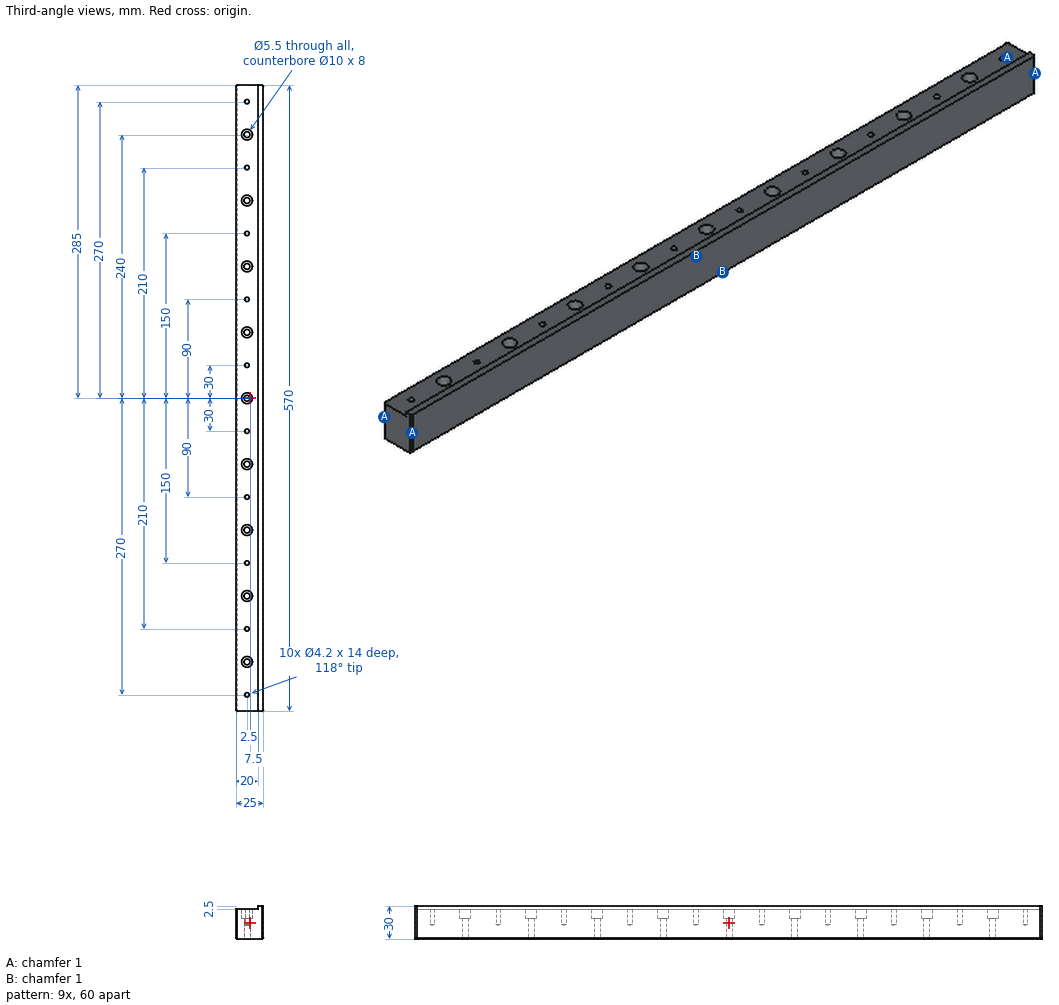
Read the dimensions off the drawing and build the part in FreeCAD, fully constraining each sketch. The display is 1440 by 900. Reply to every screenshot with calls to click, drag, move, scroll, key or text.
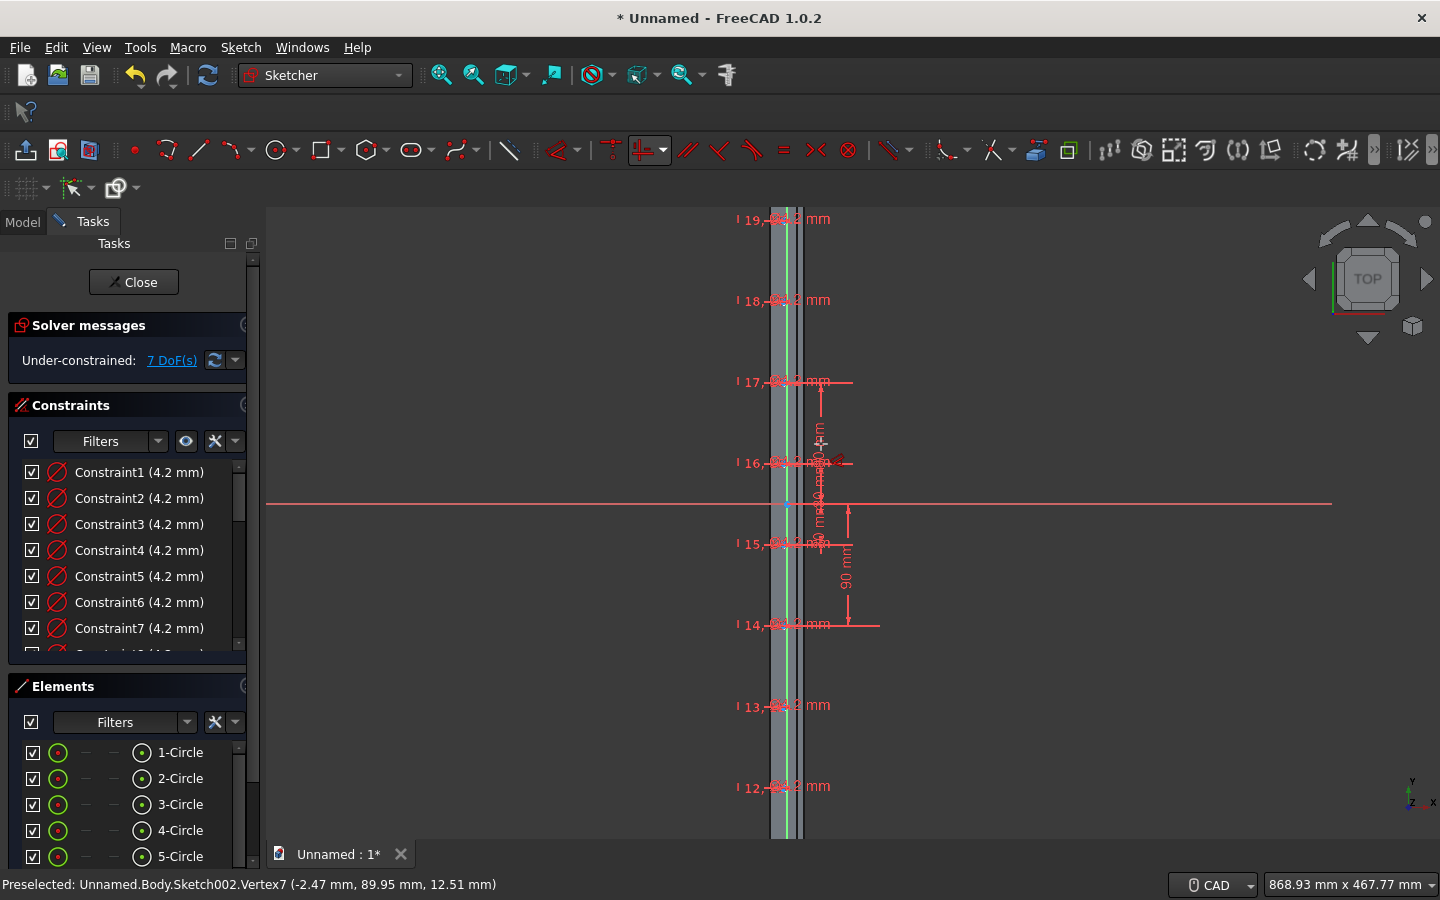
scroll(785, 546, down, 3)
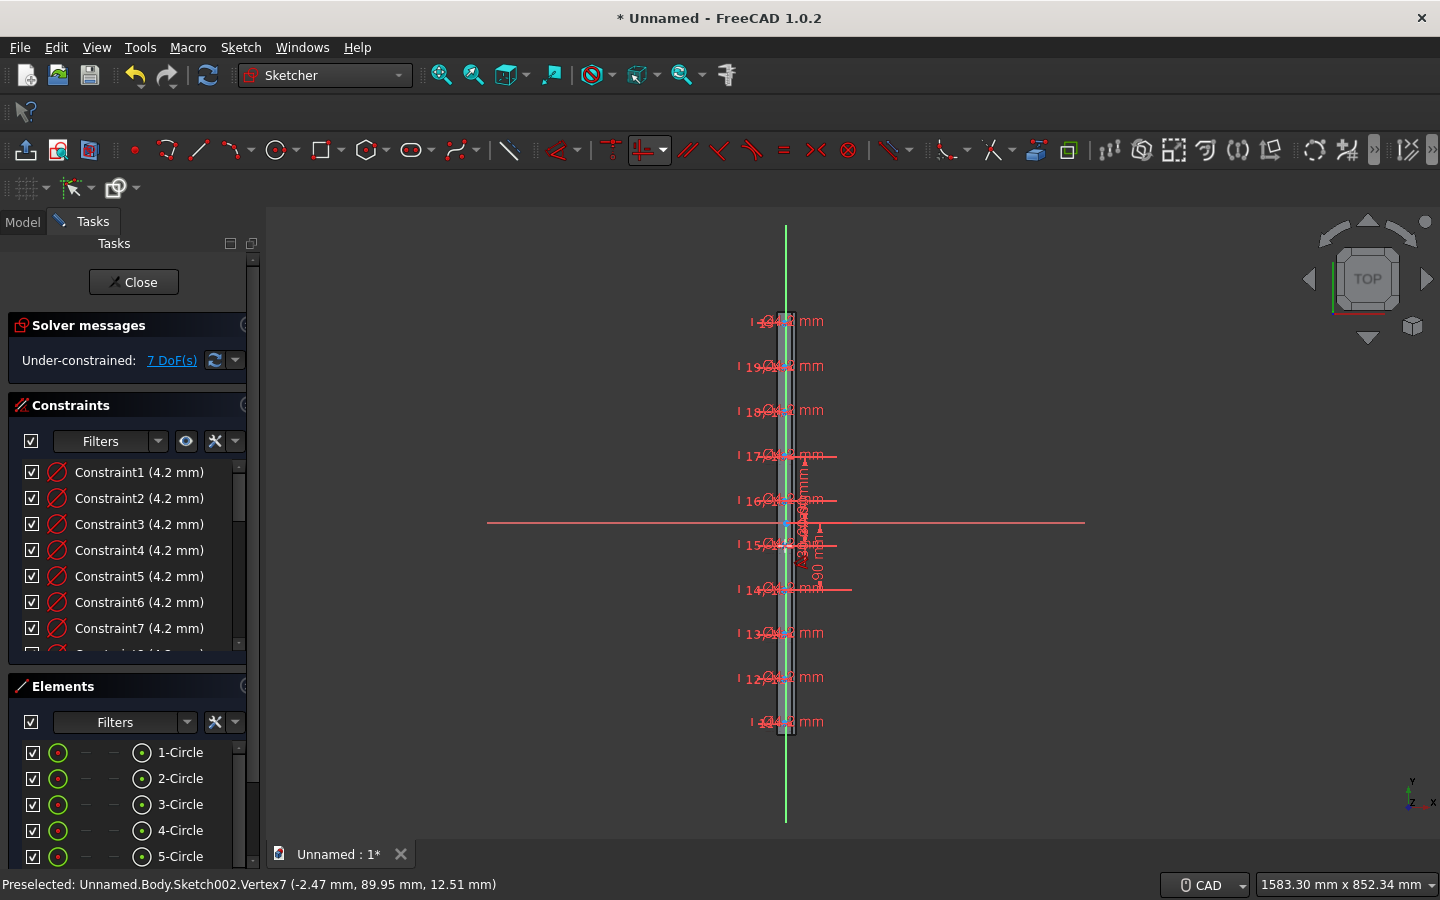
scroll(785, 724, up, 16)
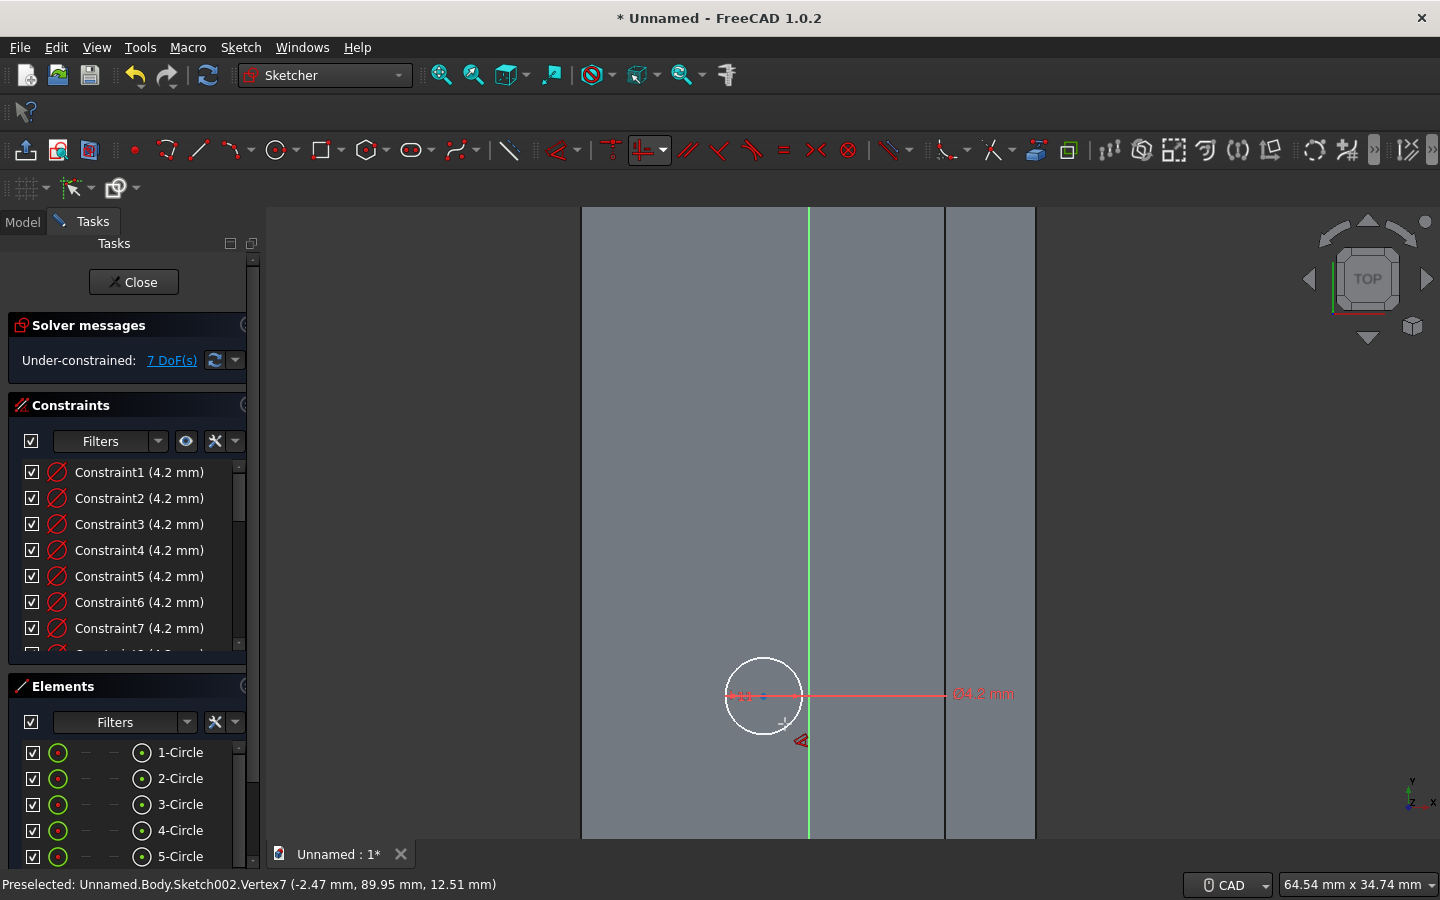
click(764, 696)
click(786, 754)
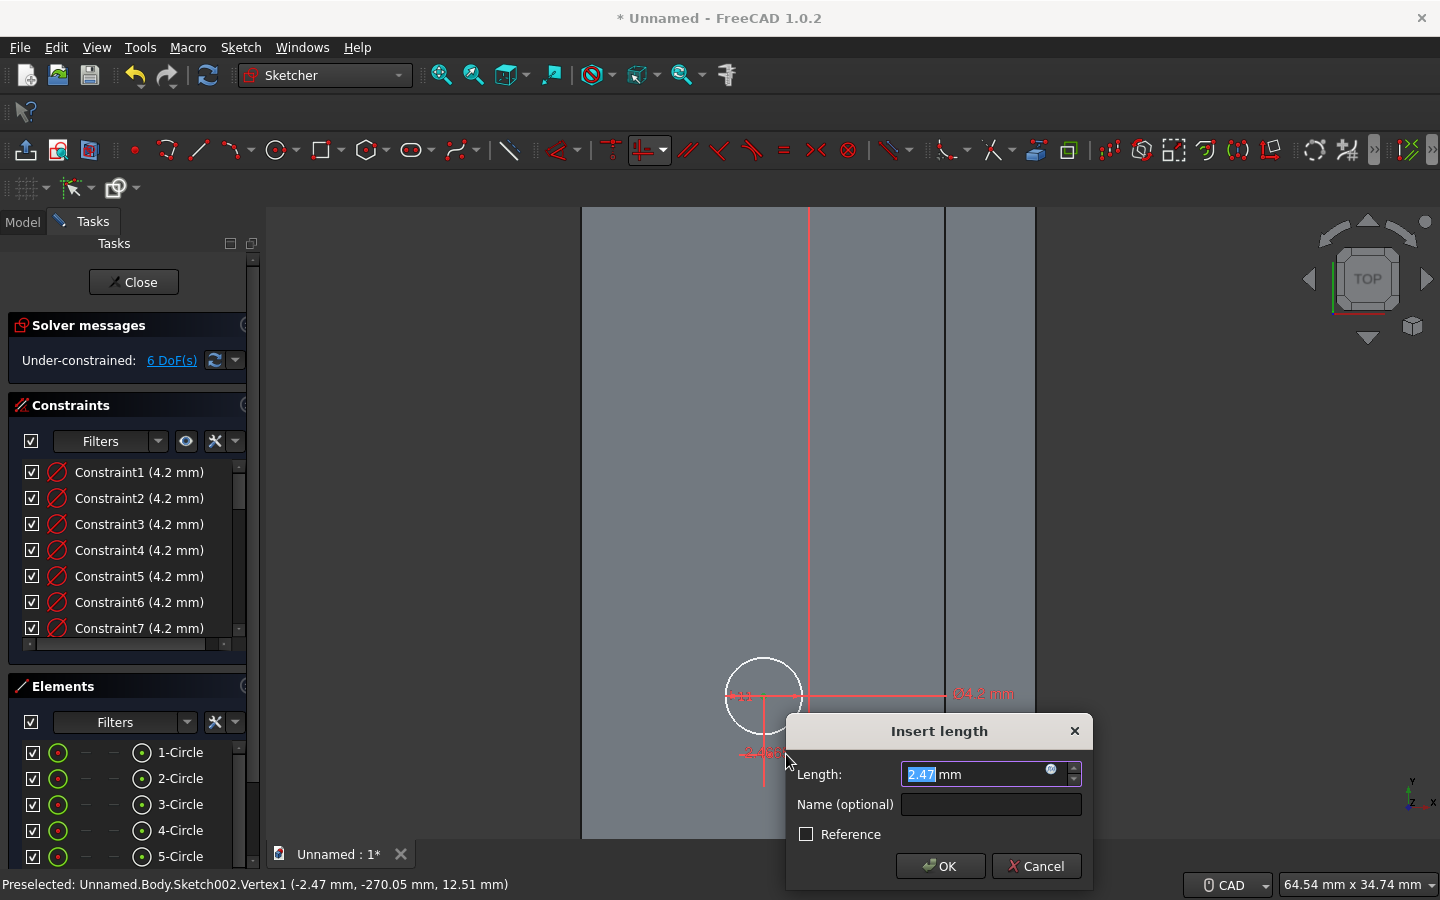
text(2.5)
key(Return)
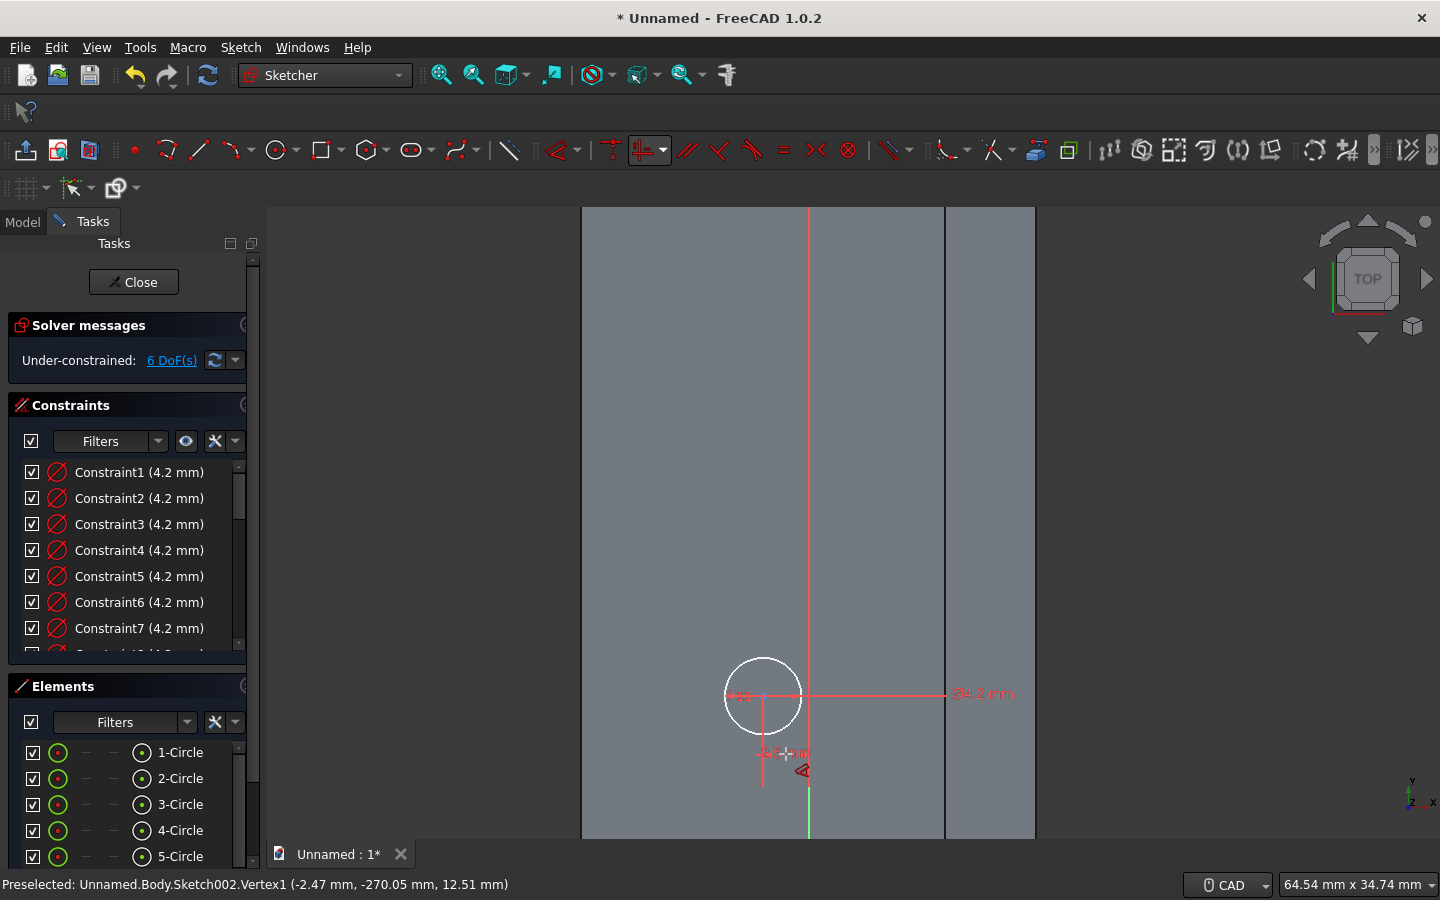
scroll(785, 771, down, 15)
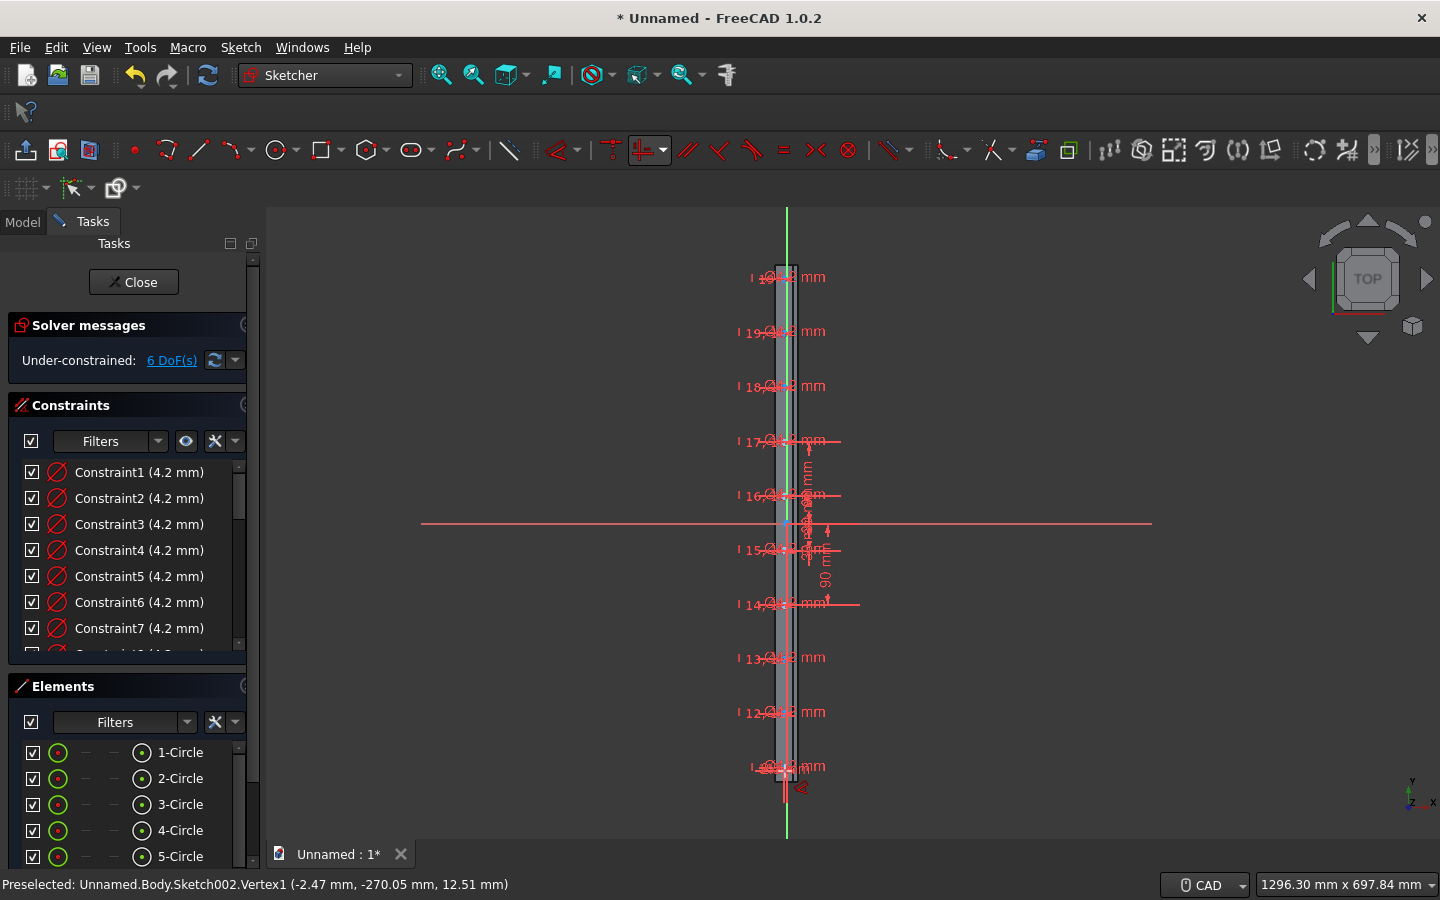
click(784, 768)
click(821, 646)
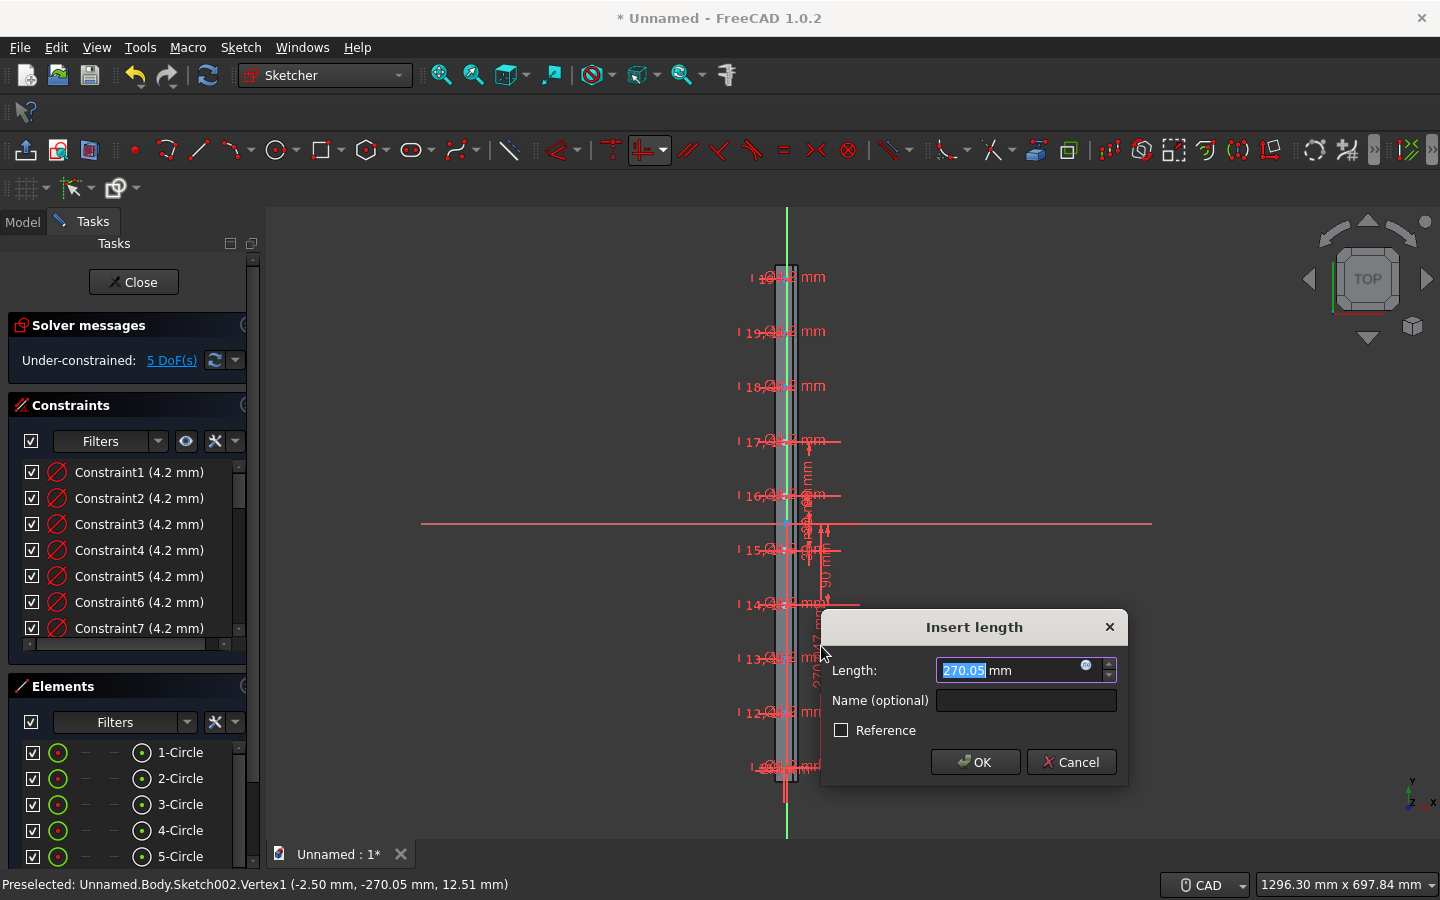
text(270)
key(Return)